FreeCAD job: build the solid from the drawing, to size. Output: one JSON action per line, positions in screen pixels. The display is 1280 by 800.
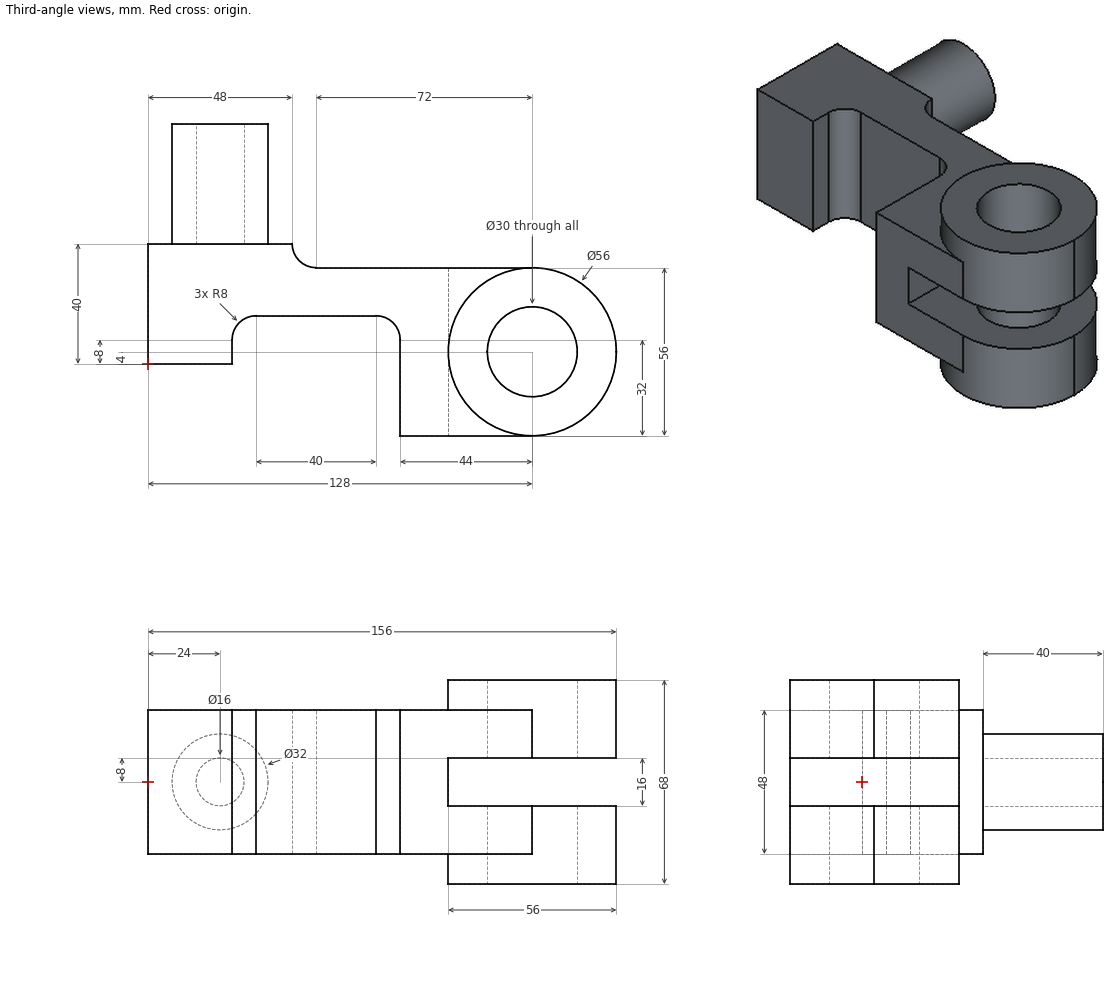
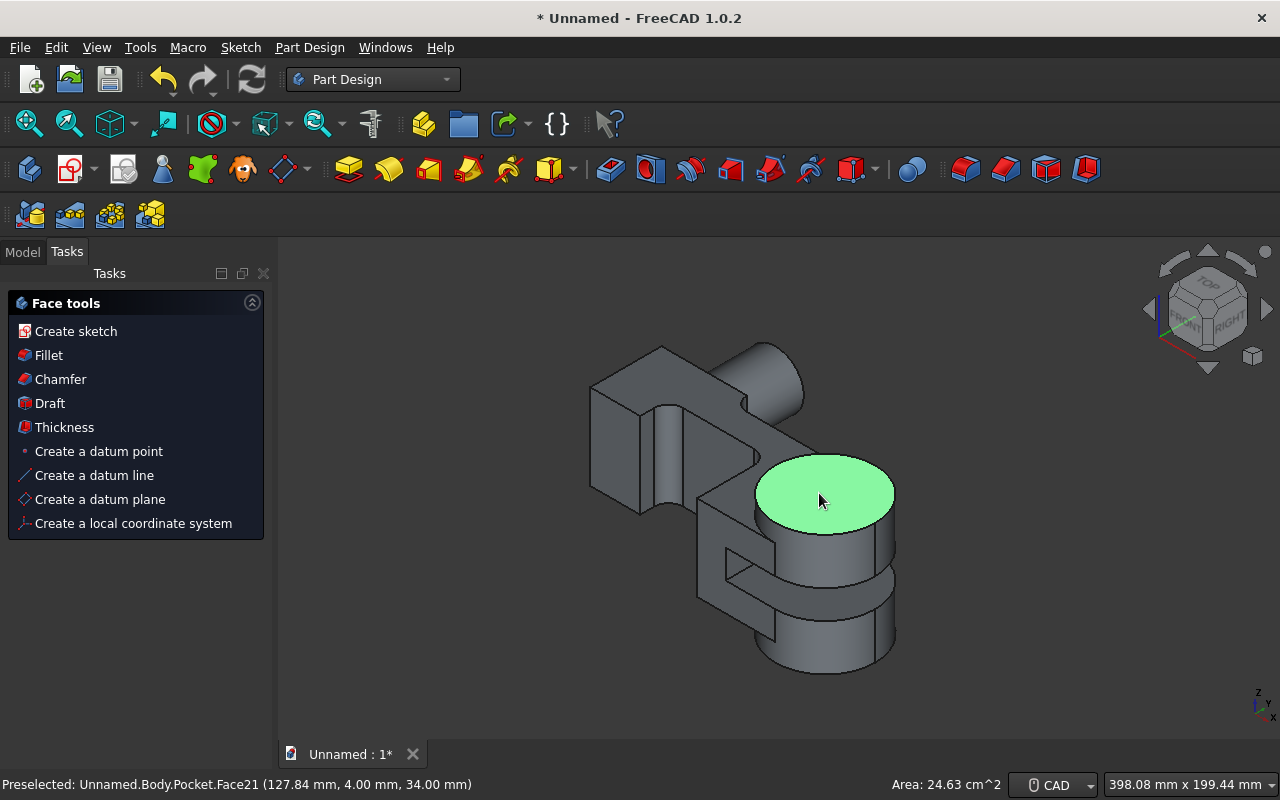
{"action": "left_click", "coordinate": [70, 170]}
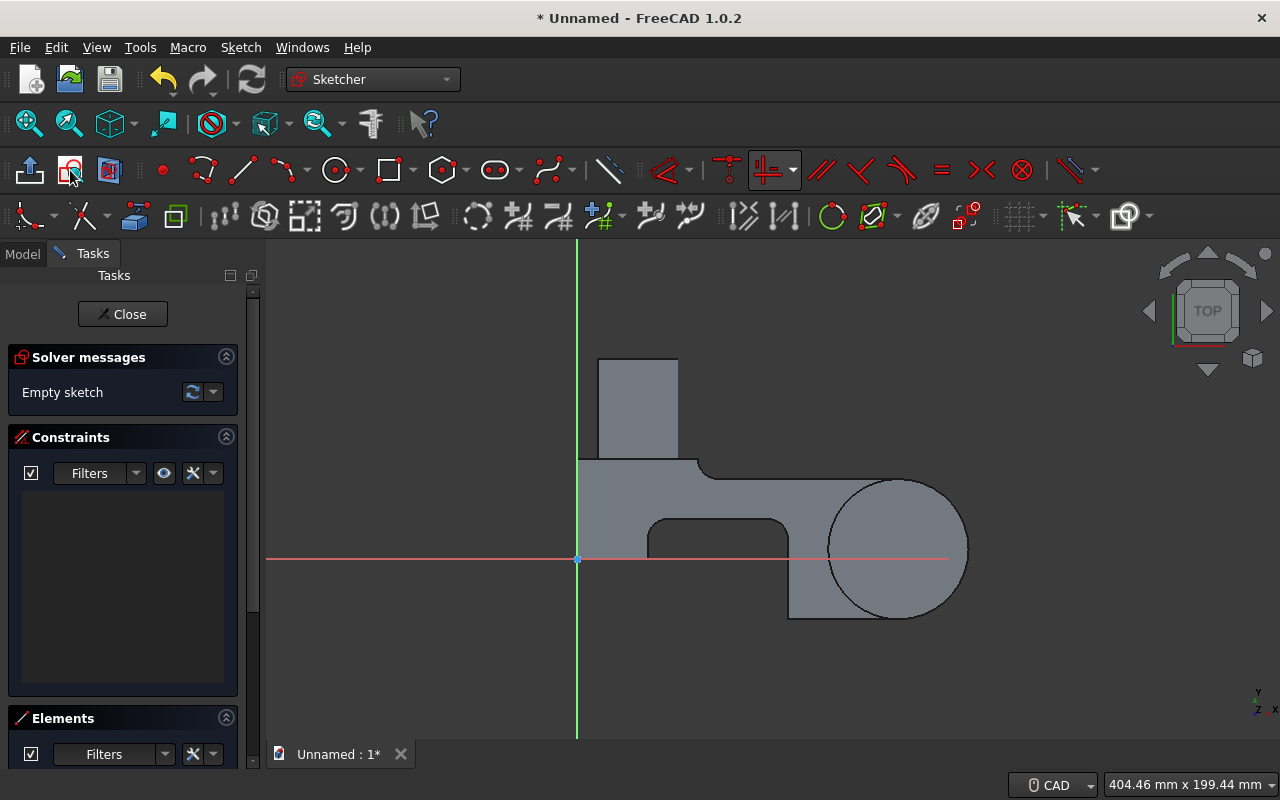
{"action": "scroll", "coordinate": [962, 569], "scroll_direction": "up", "scroll_amount": 7}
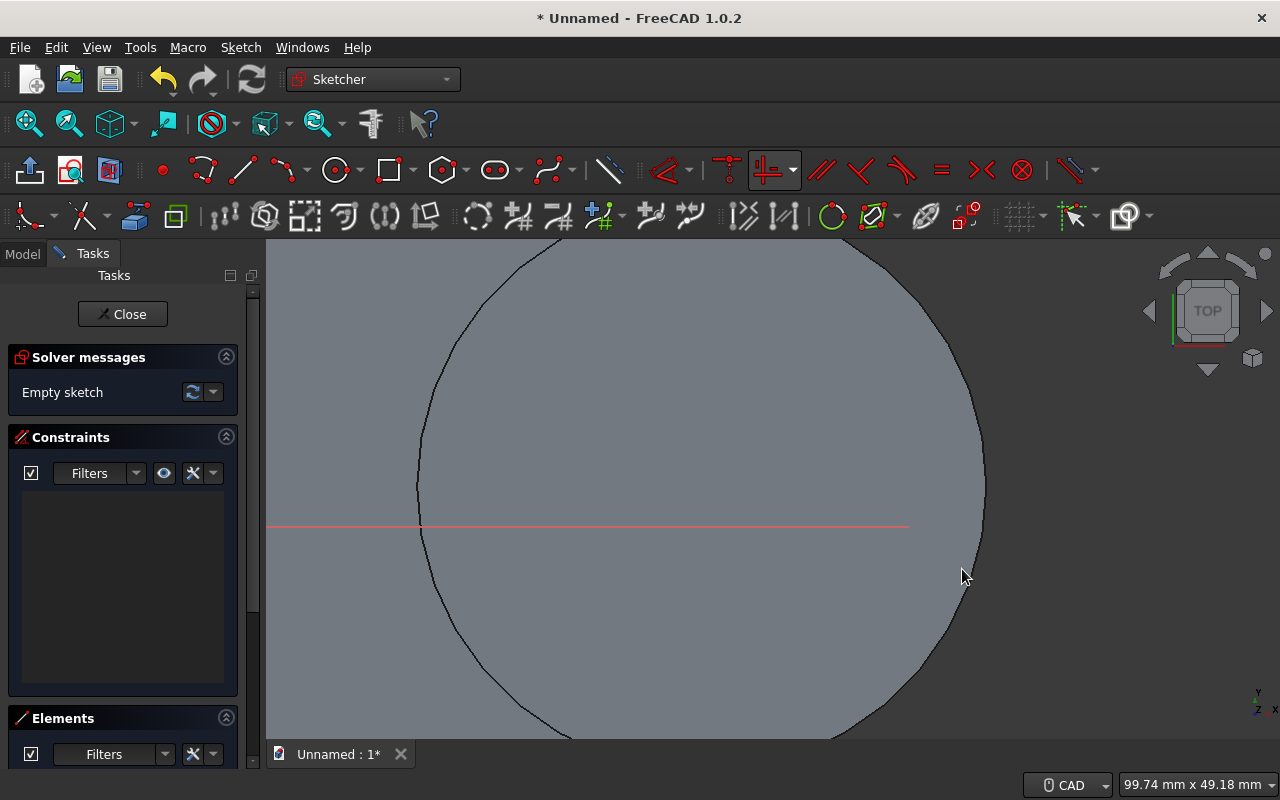
{"action": "key", "text": "g c"}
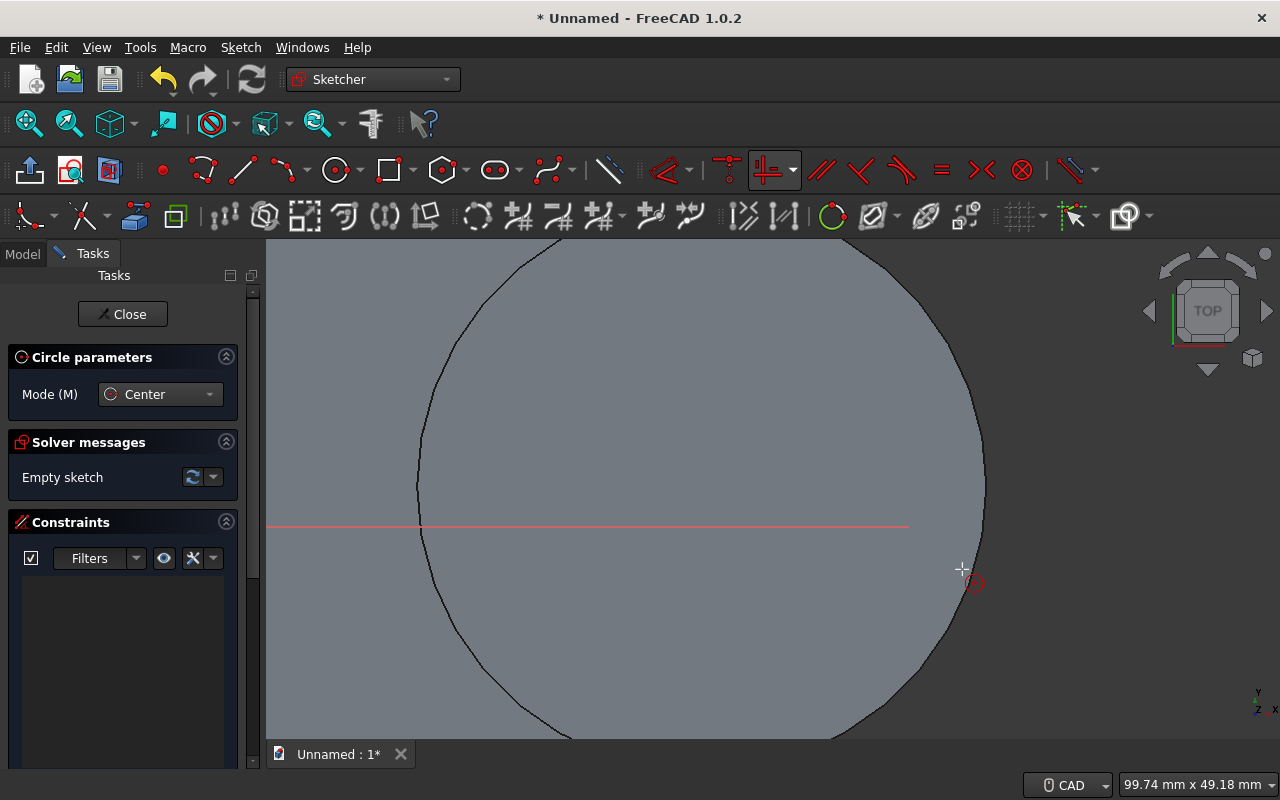
{"action": "left_click", "coordinate": [702, 487]}
{"action": "mouse_move", "coordinate": [810, 379]}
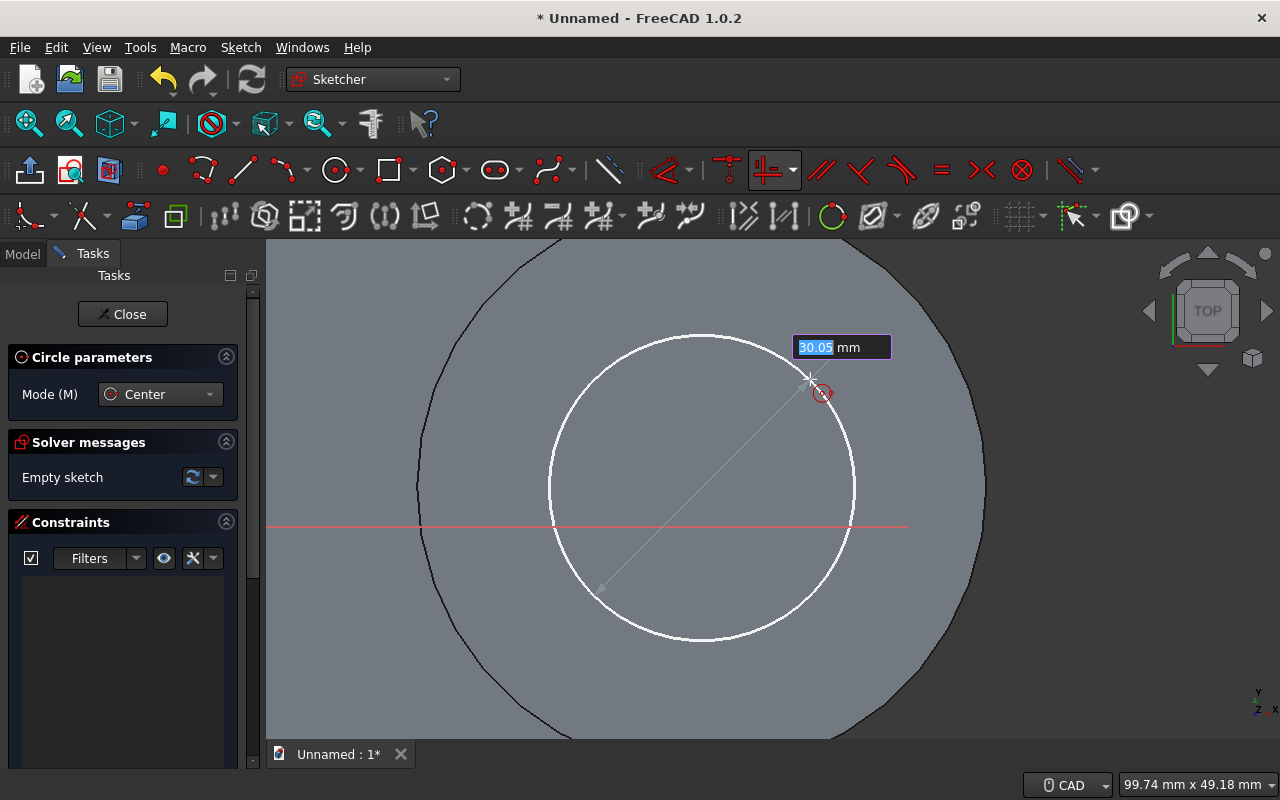
{"action": "type", "text": "30"}
{"action": "key", "text": "Return"}
{"action": "key", "text": "Escape"}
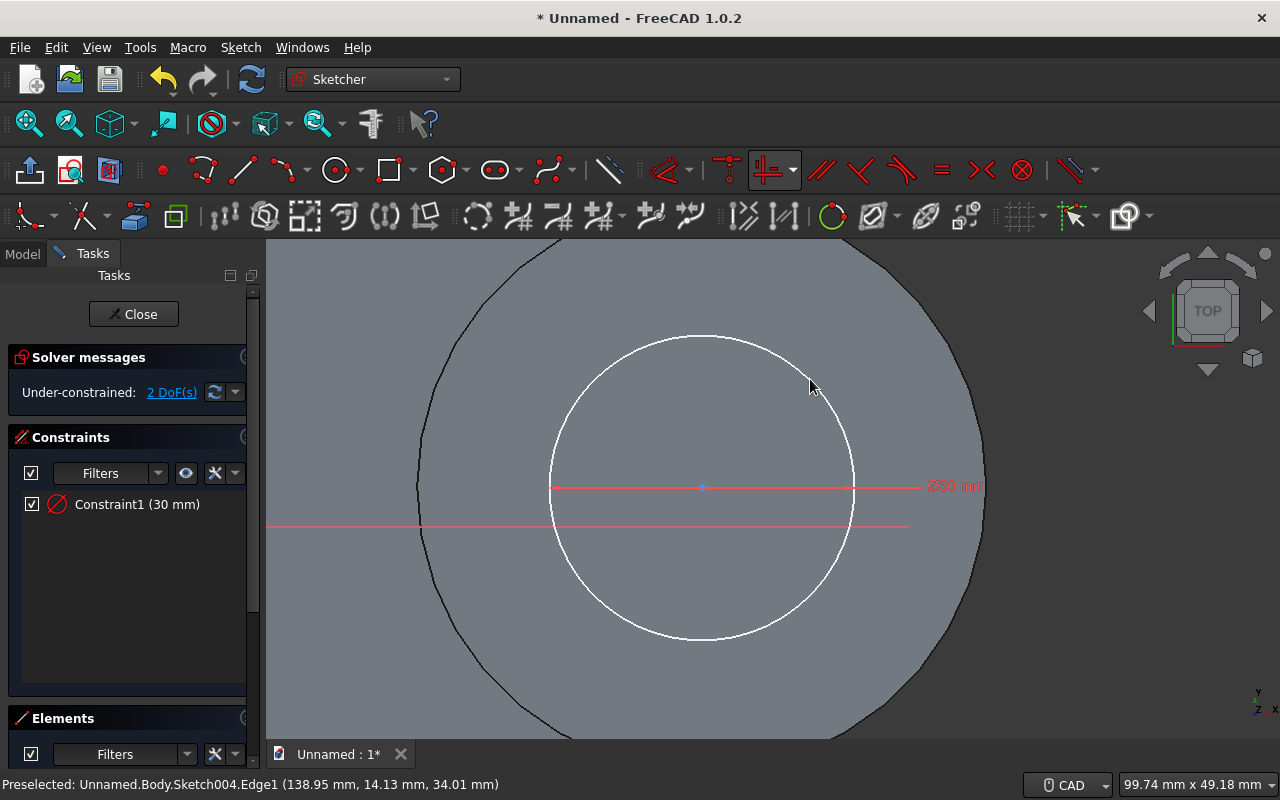
{"action": "key", "text": "d"}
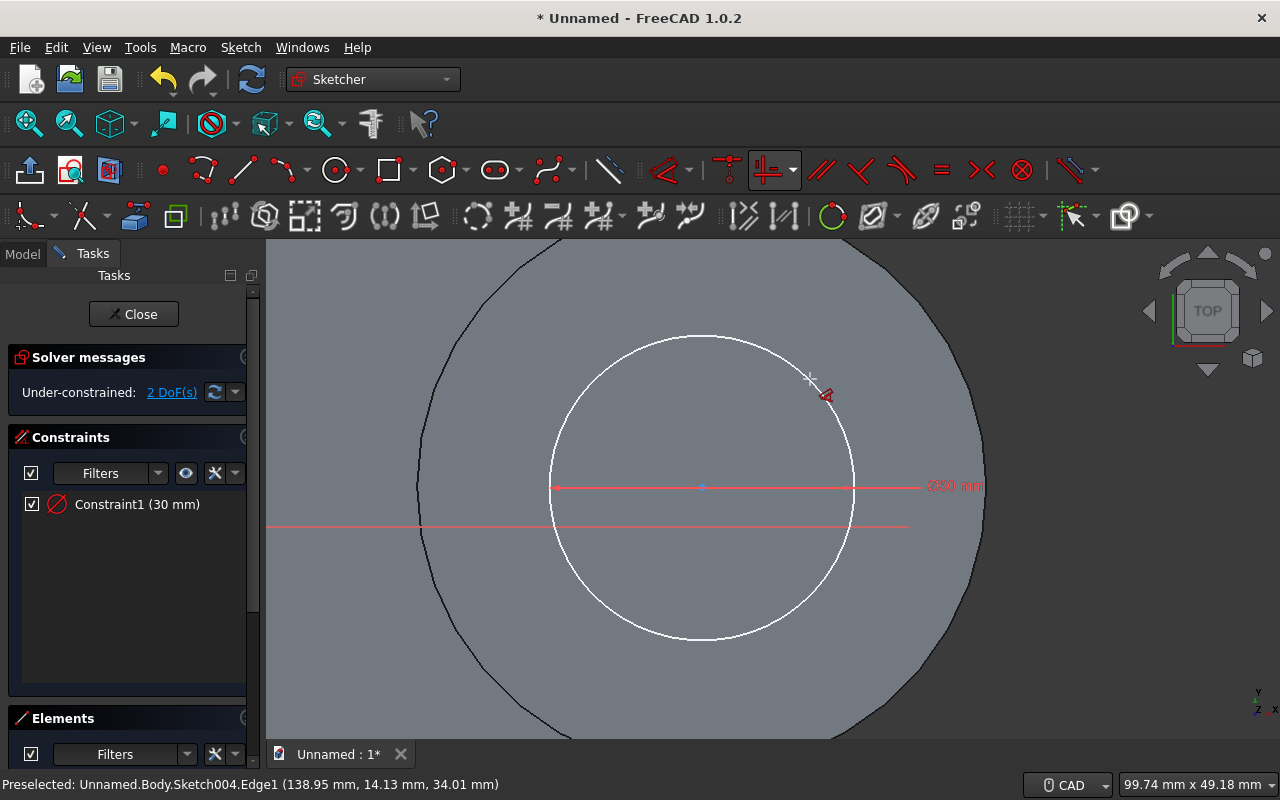
{"action": "left_click", "coordinate": [702, 488]}
{"action": "left_click", "coordinate": [736, 508]}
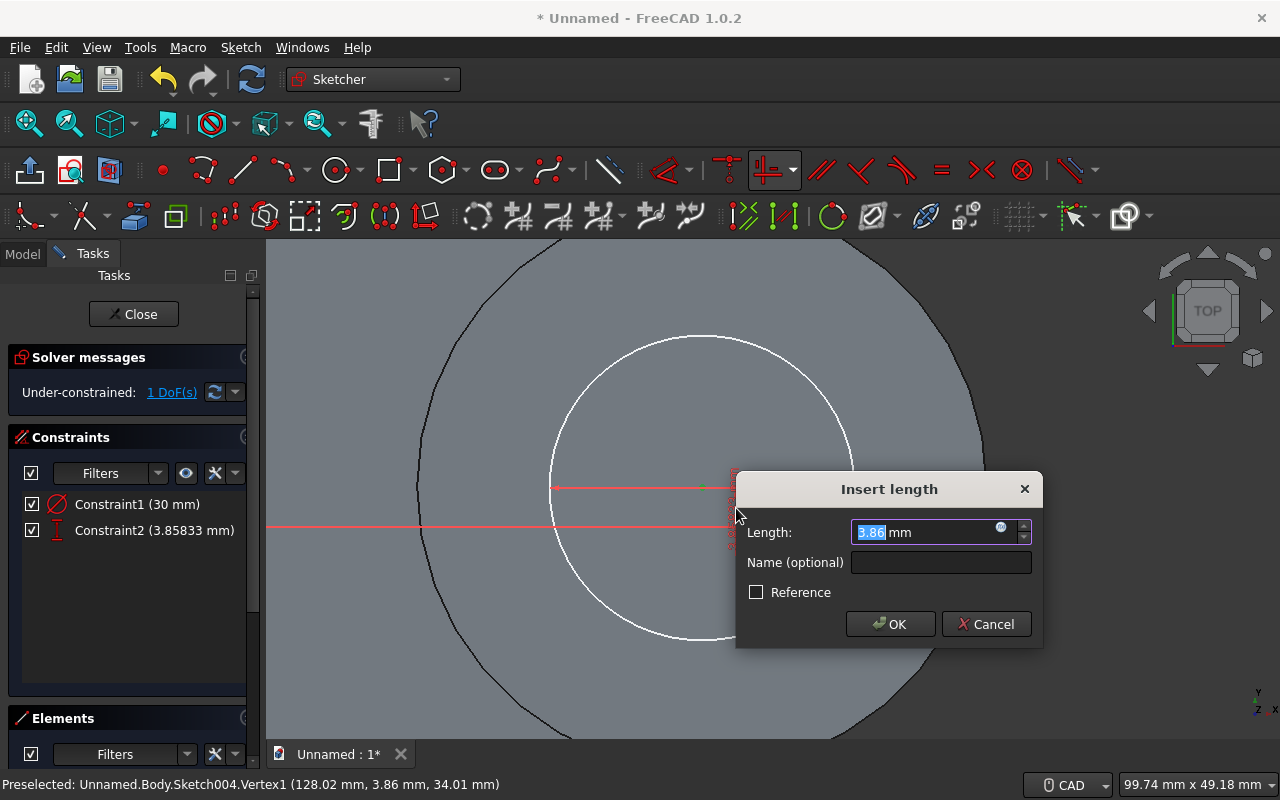
{"action": "type", "text": "4"}
{"action": "key", "text": "Return"}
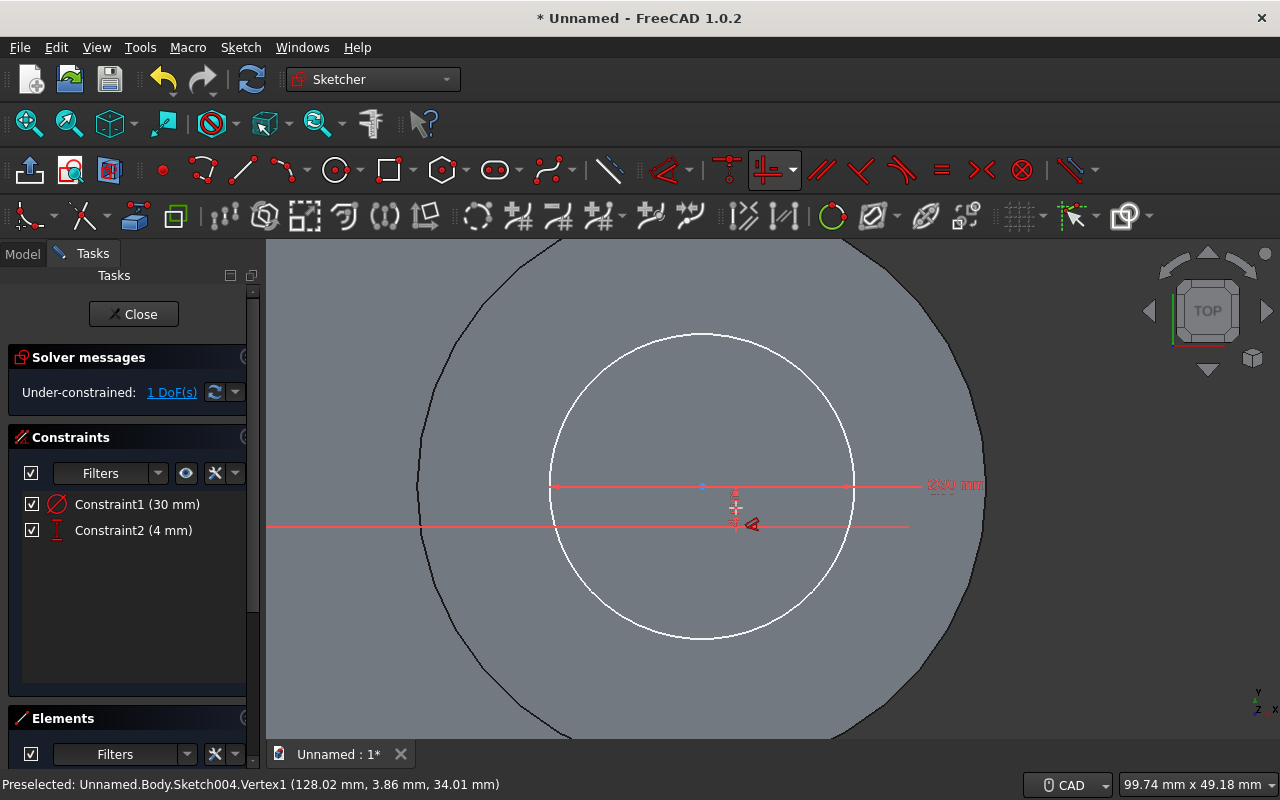
{"action": "left_click", "coordinate": [702, 487]}
{"action": "left_click", "coordinate": [498, 561]}